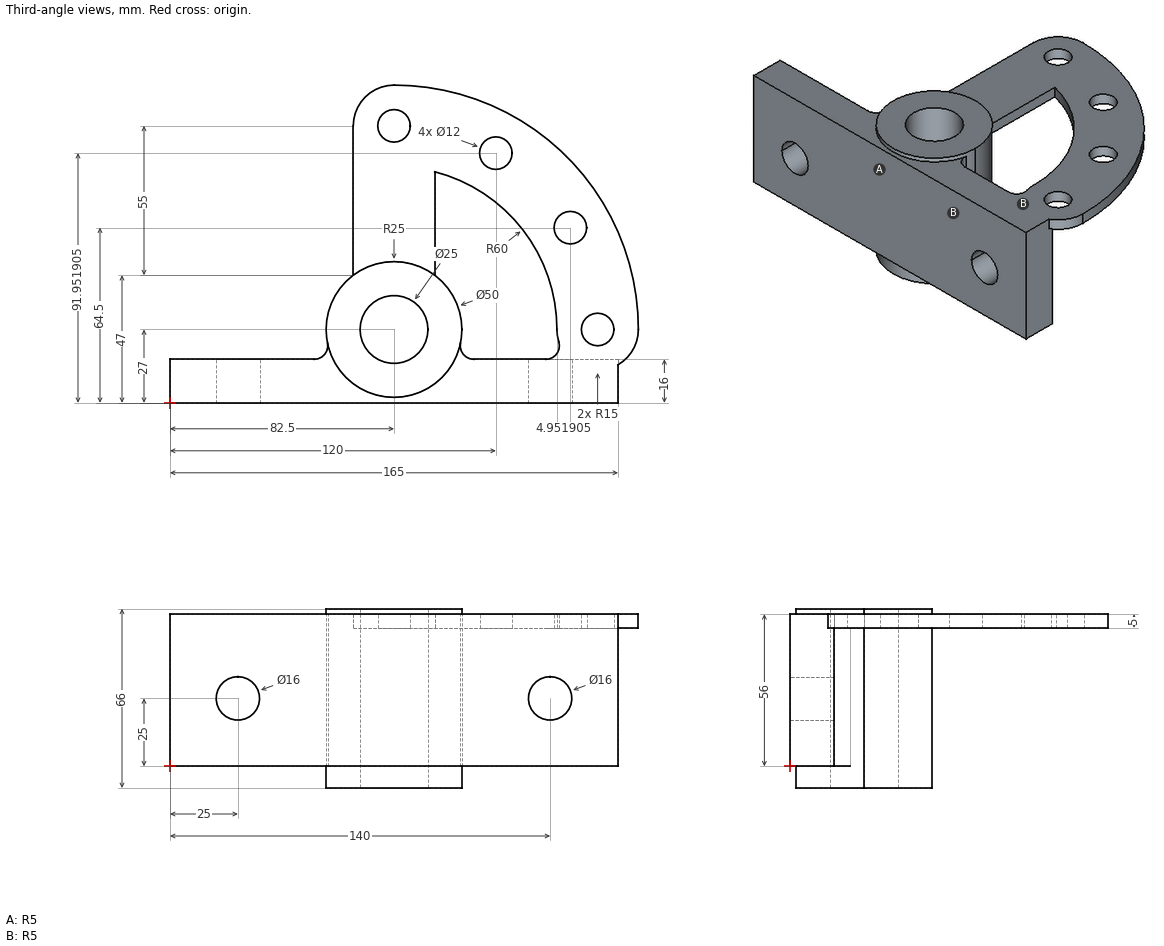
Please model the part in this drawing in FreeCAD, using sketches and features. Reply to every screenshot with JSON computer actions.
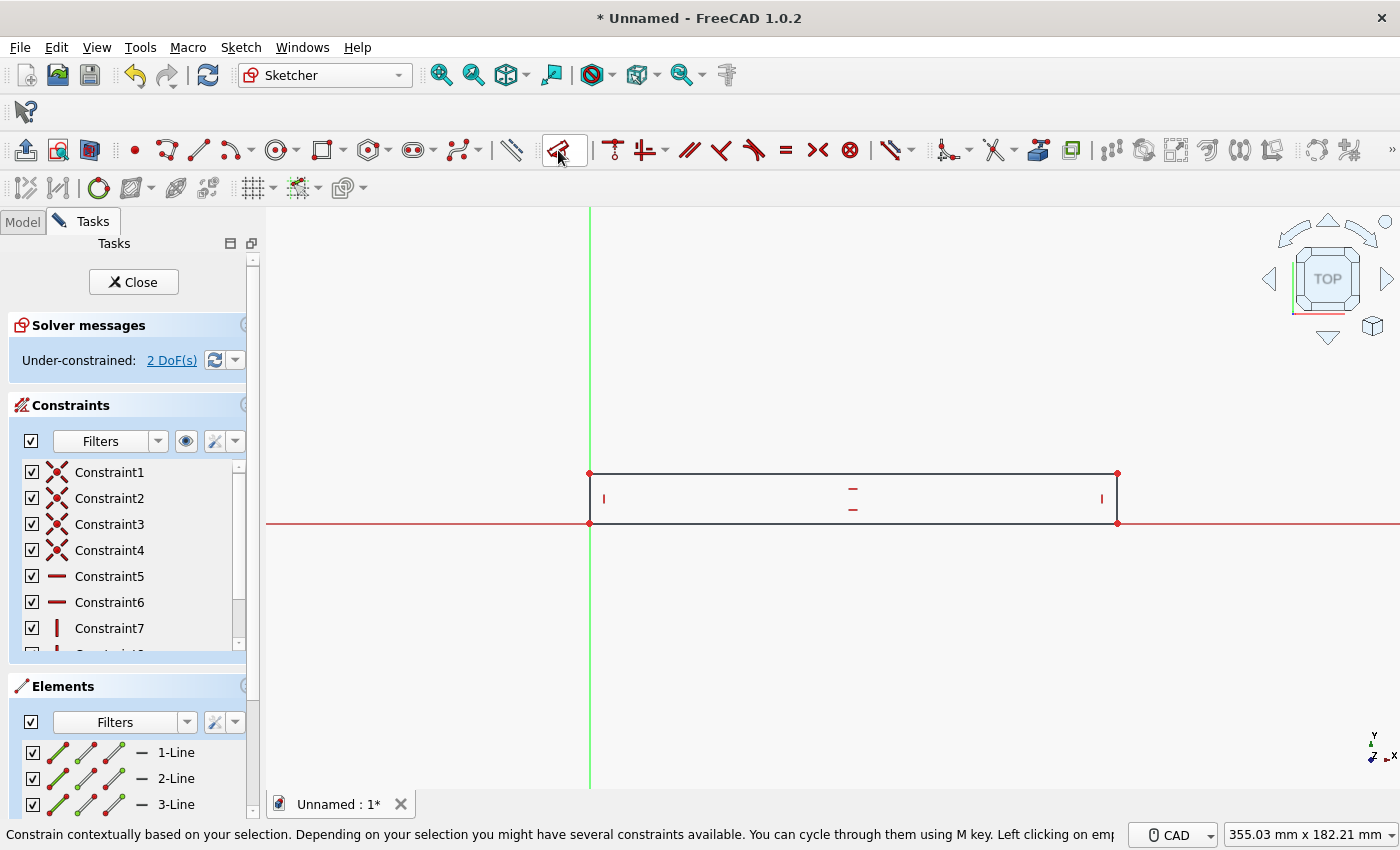
{"action": "left_click", "coordinate": [1117, 509]}
{"action": "left_click", "coordinate": [1151, 499]}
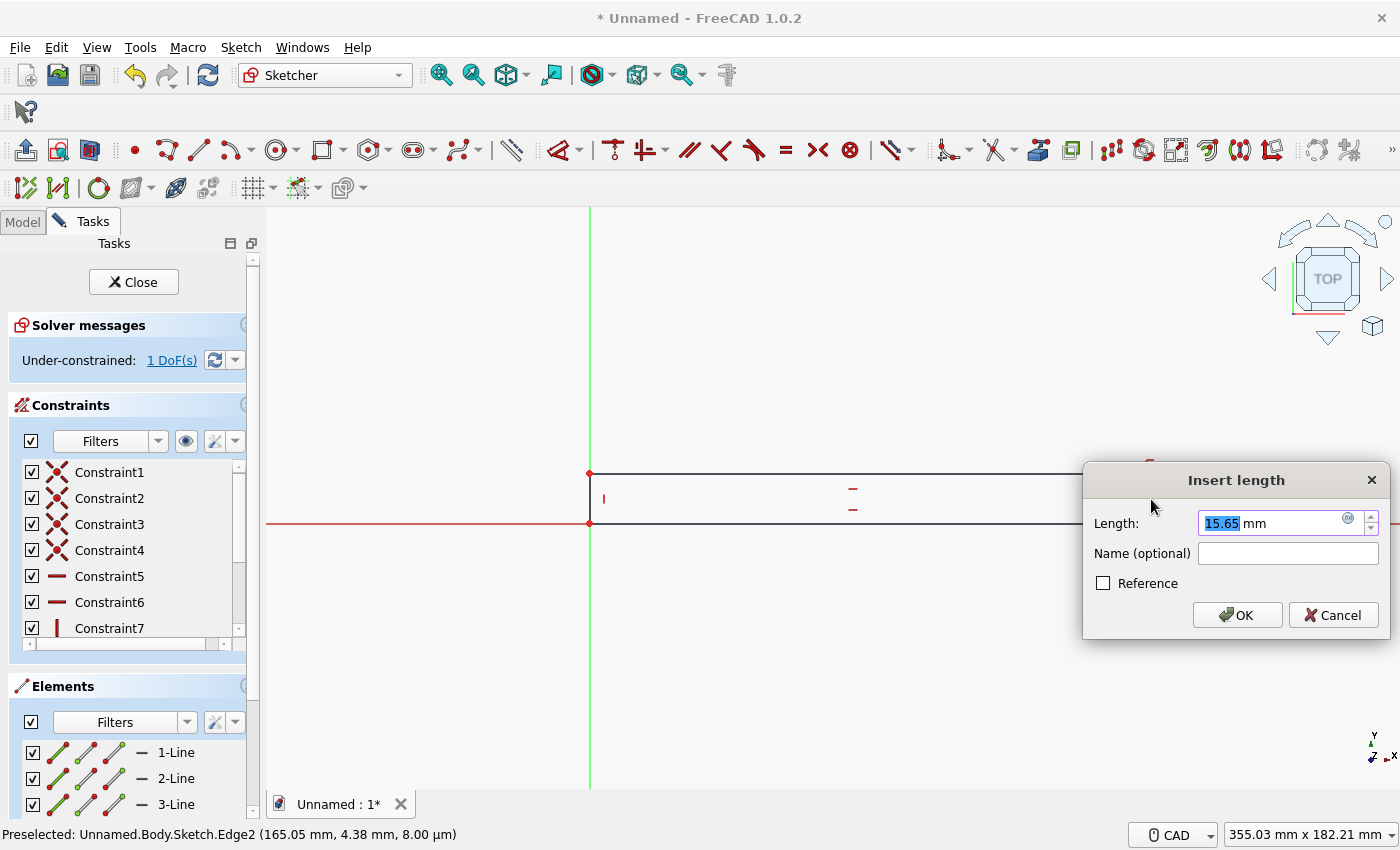
{"action": "type", "text": "16"}
{"action": "key", "text": "Return"}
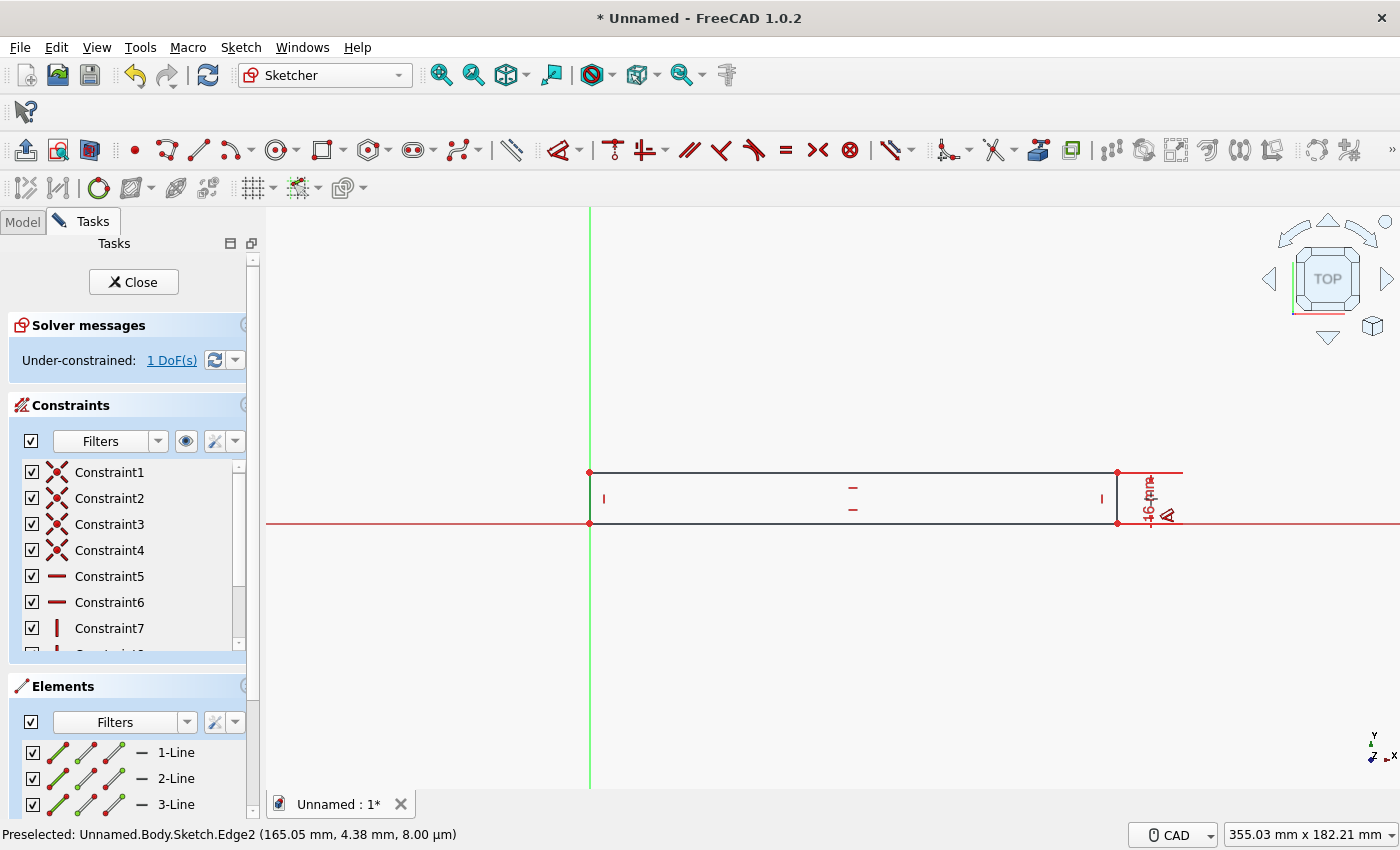
{"action": "left_click", "coordinate": [748, 524]}
{"action": "left_click", "coordinate": [853, 558]}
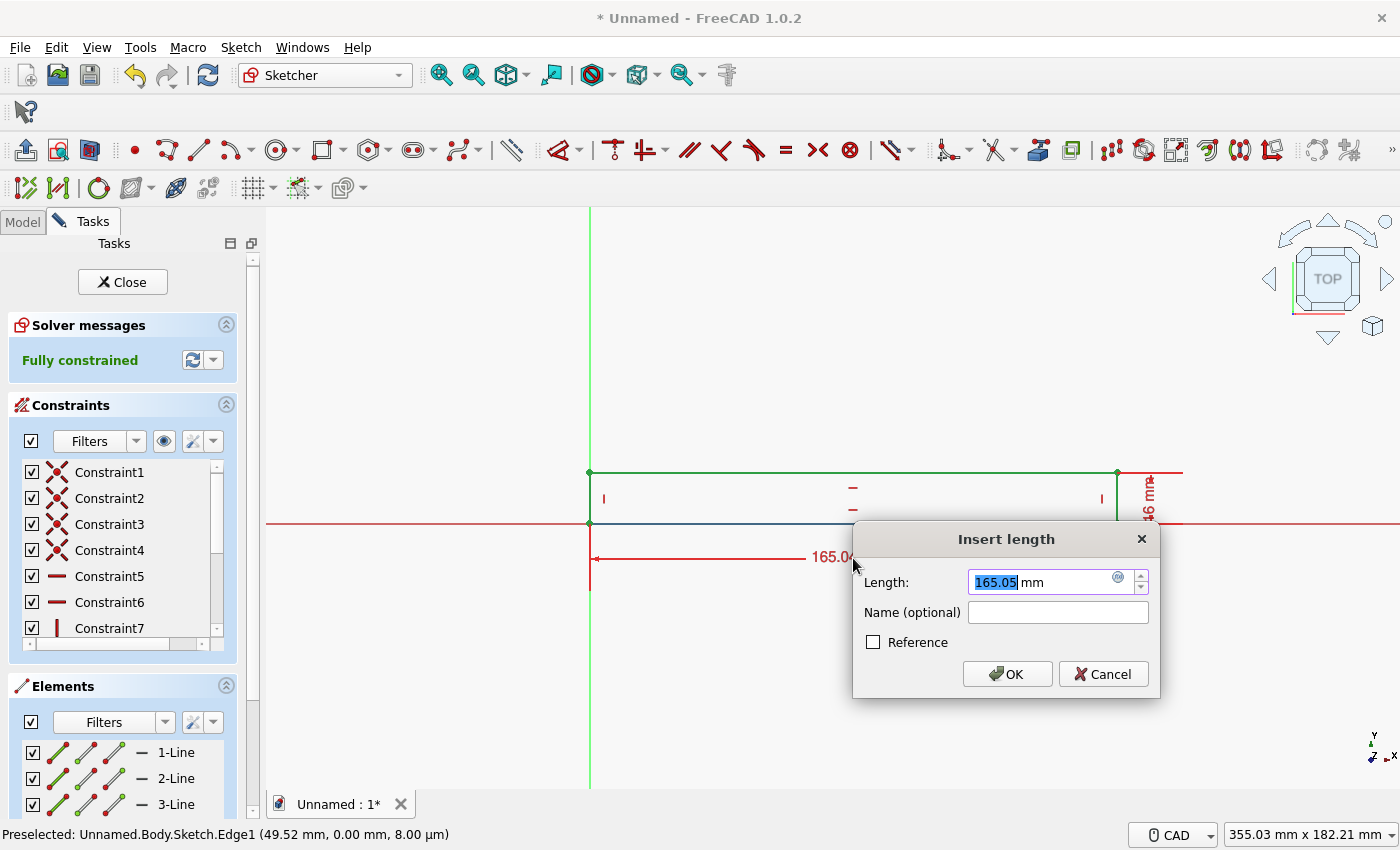
{"action": "type", "text": "165"}
{"action": "key", "text": "Return"}
{"action": "key", "text": "Escape"}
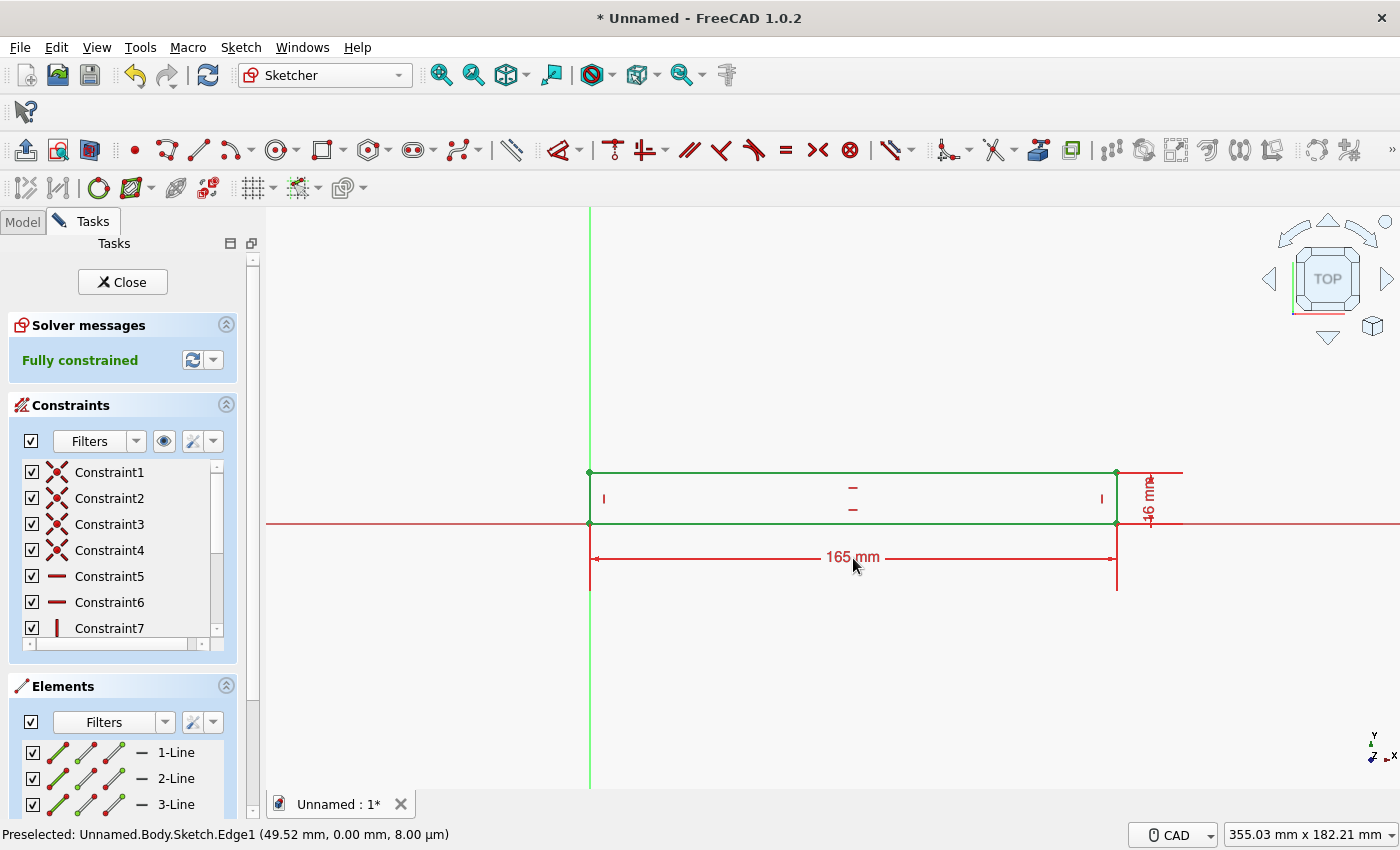
{"action": "left_click", "coordinate": [123, 282]}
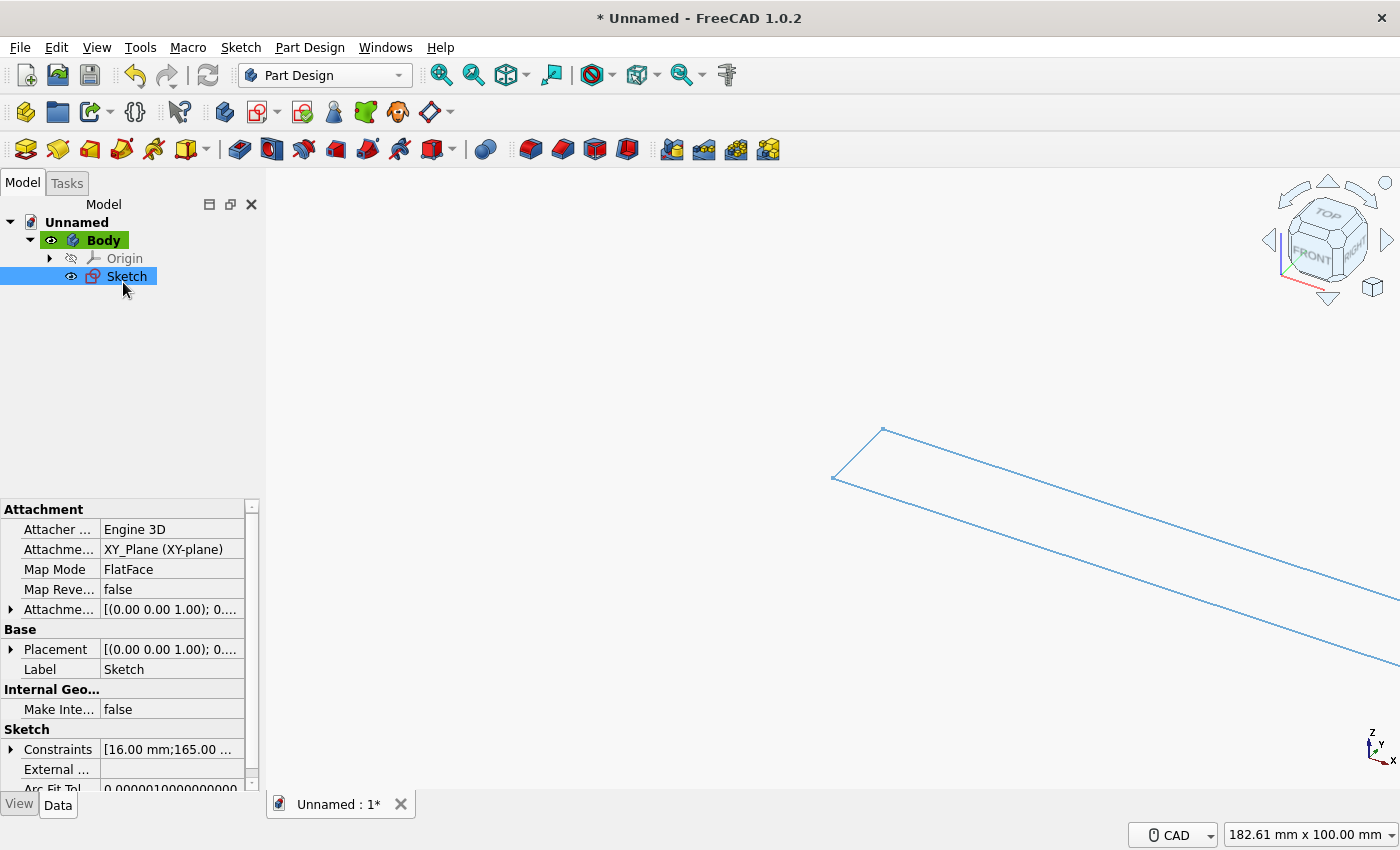
{"action": "left_click", "coordinate": [26, 150]}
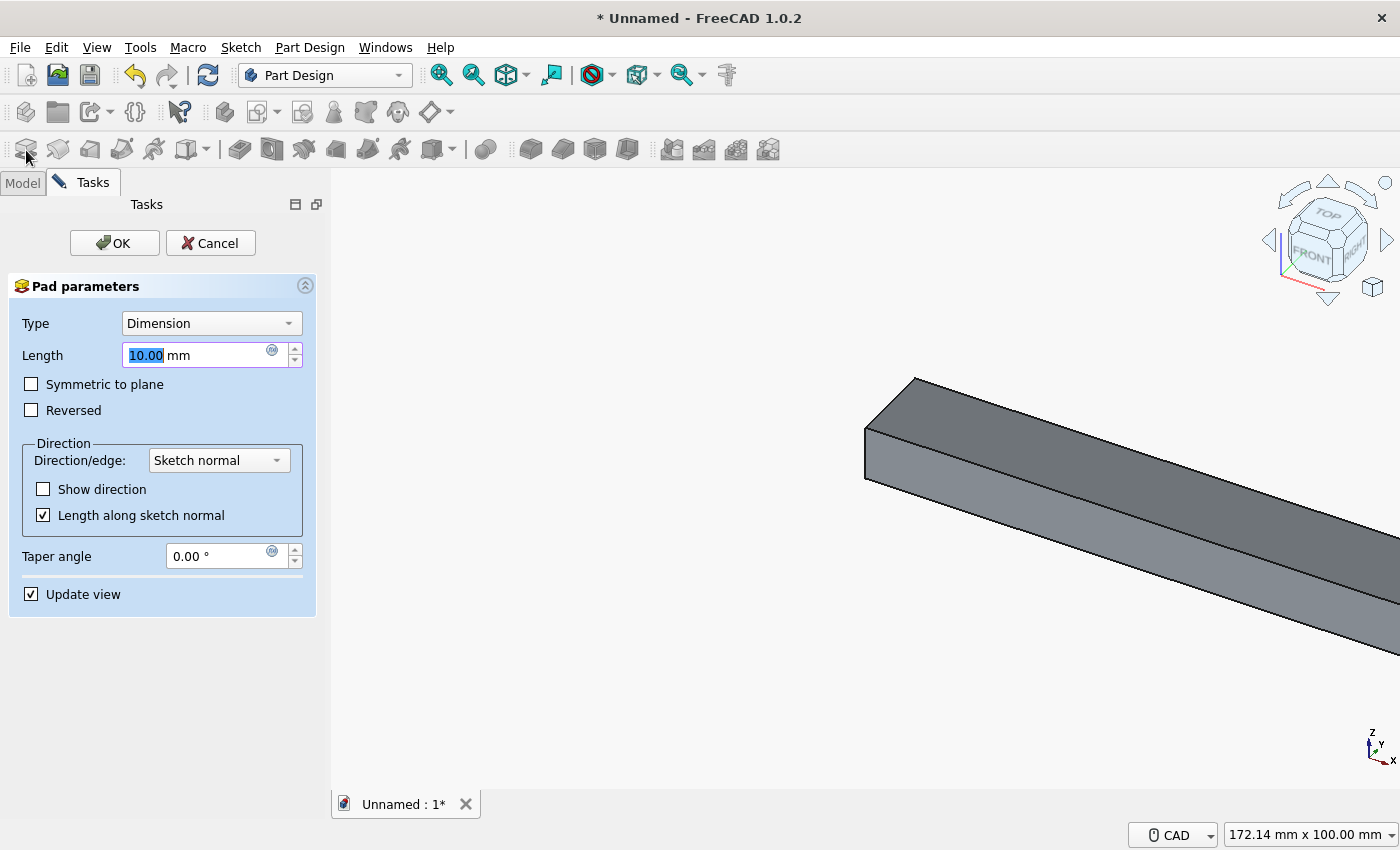
{"action": "type", "text": "56"}
{"action": "key", "text": "Tab"}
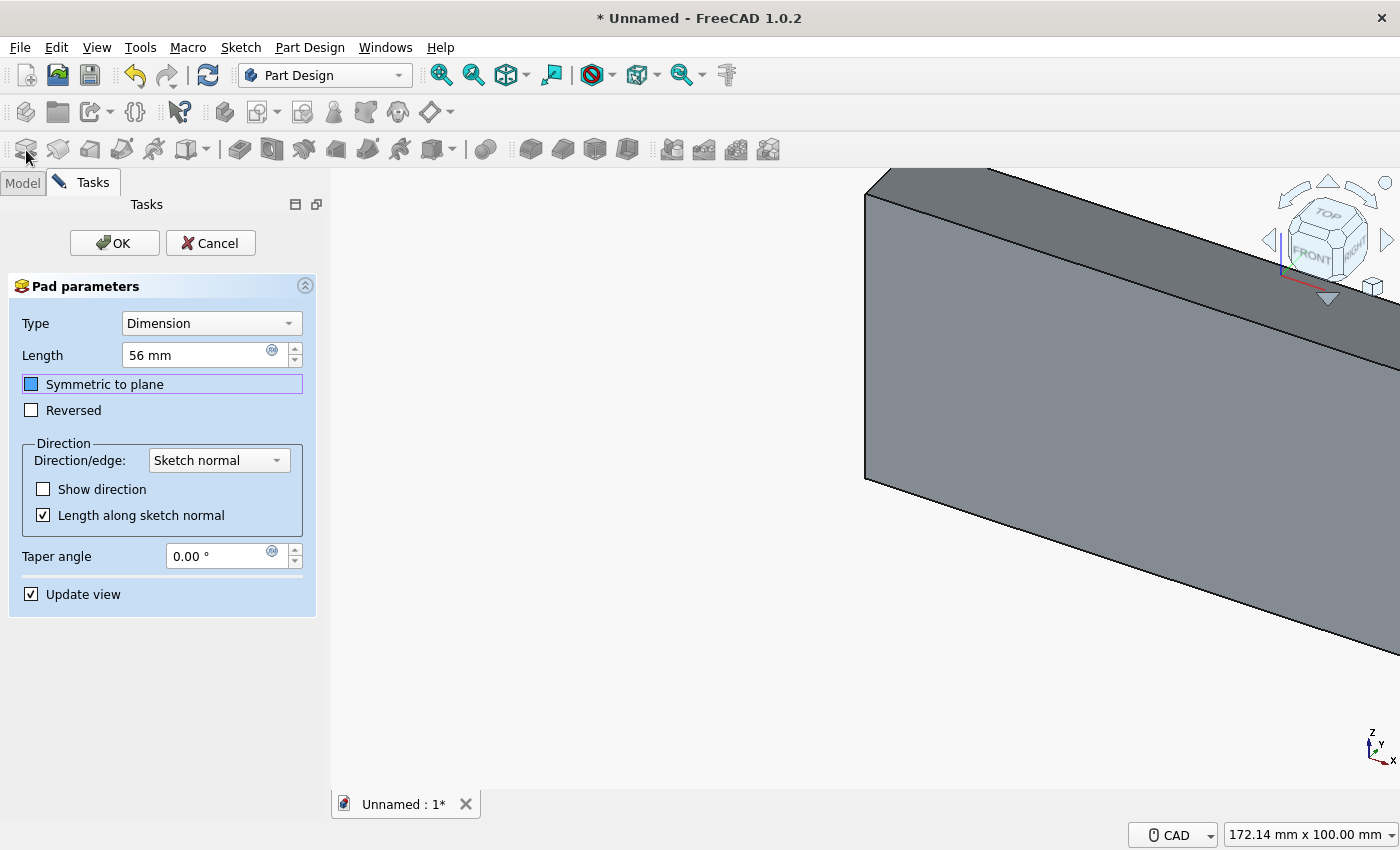
{"action": "left_click", "coordinate": [115, 243]}